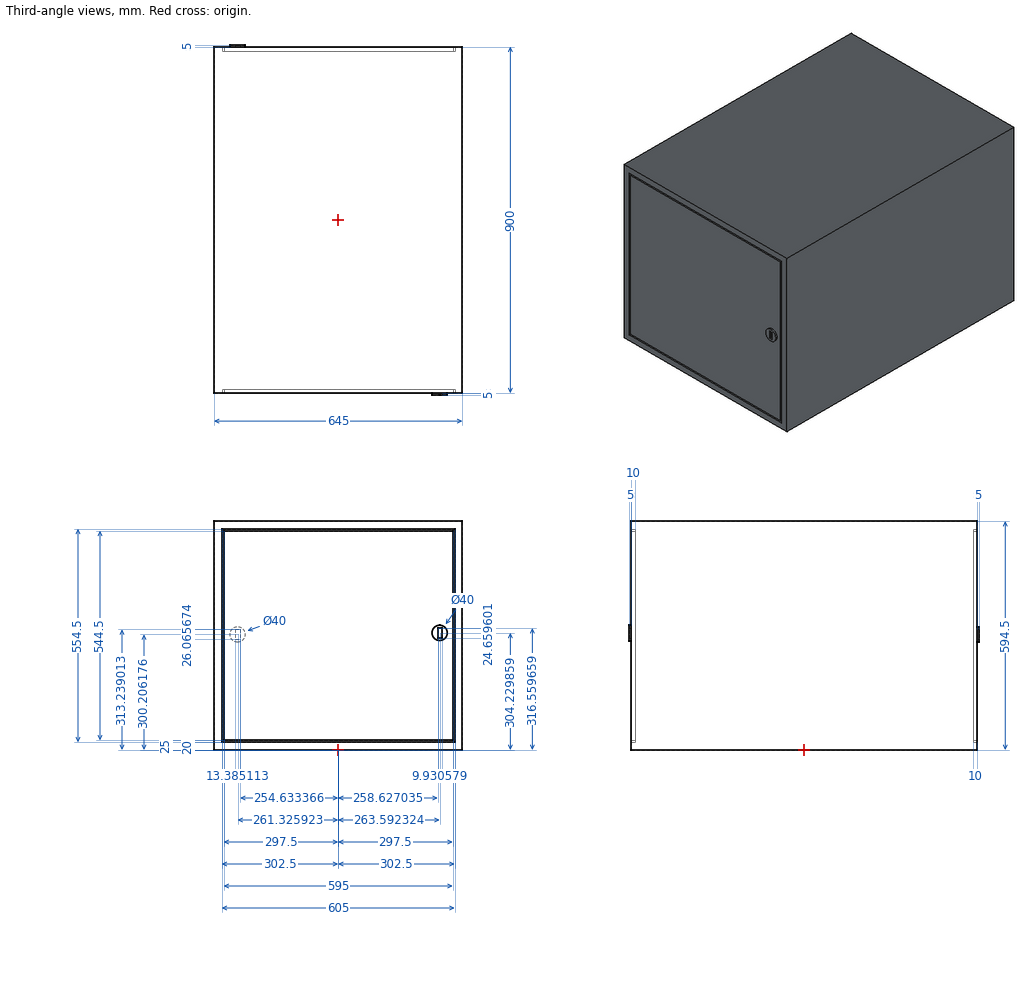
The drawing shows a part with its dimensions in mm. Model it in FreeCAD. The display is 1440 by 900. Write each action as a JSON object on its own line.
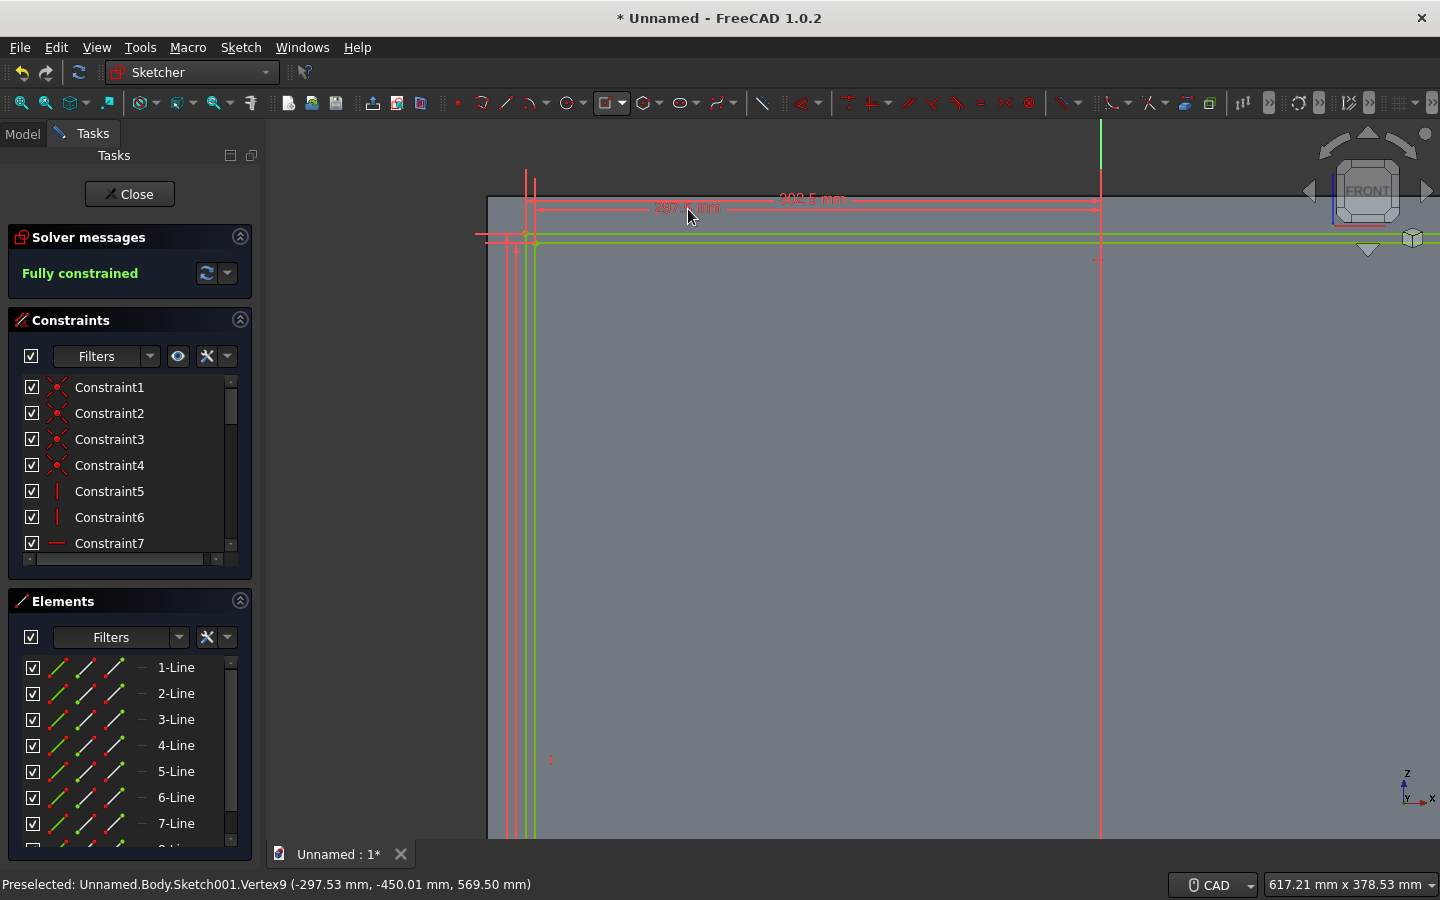
{"action": "left_click", "coordinate": [130, 194]}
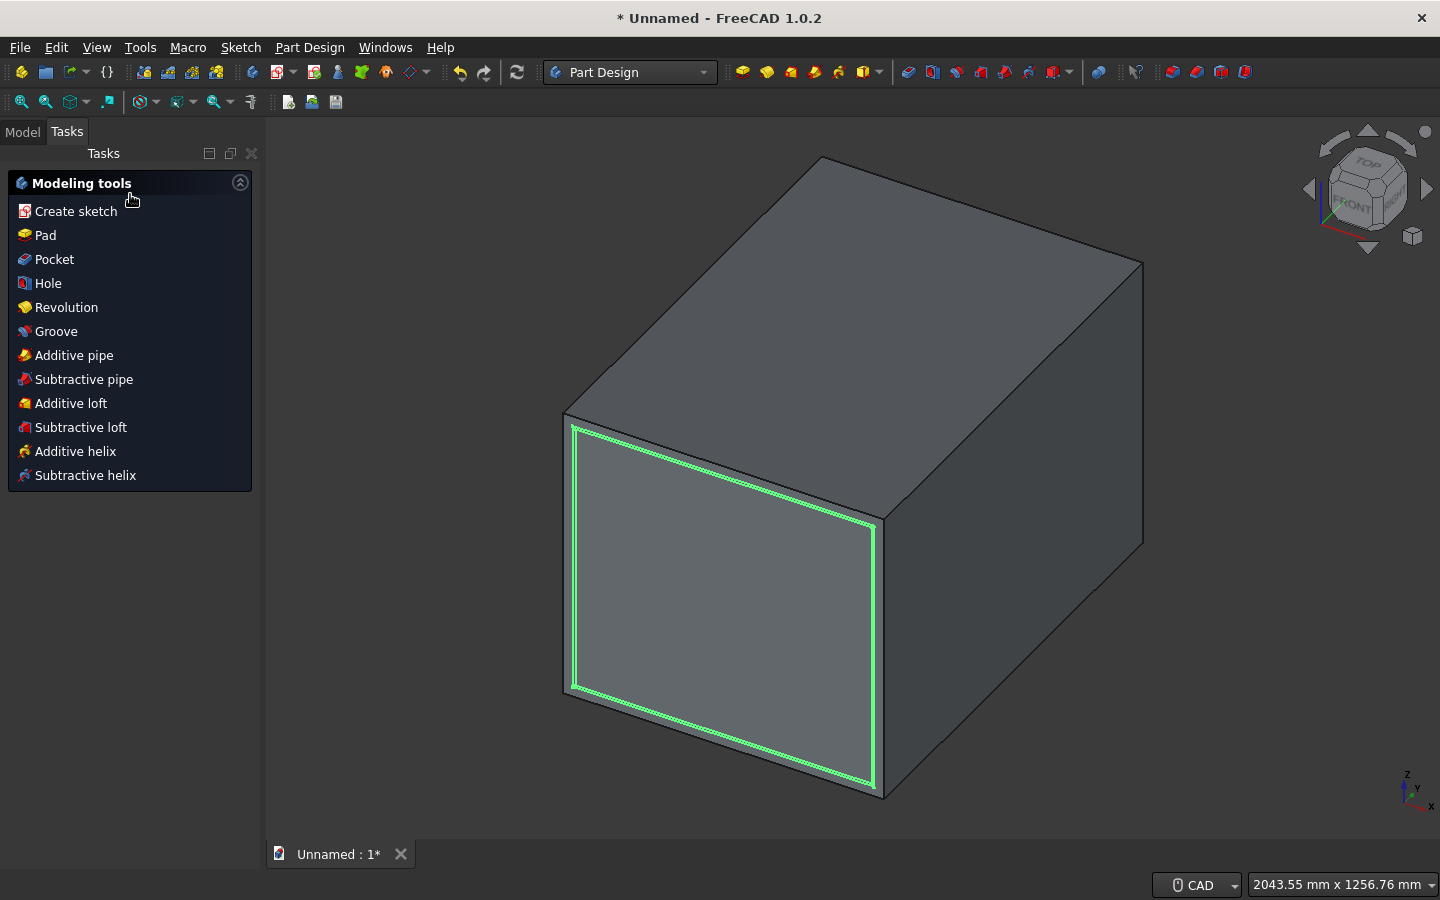
{"action": "left_click", "coordinate": [910, 72]}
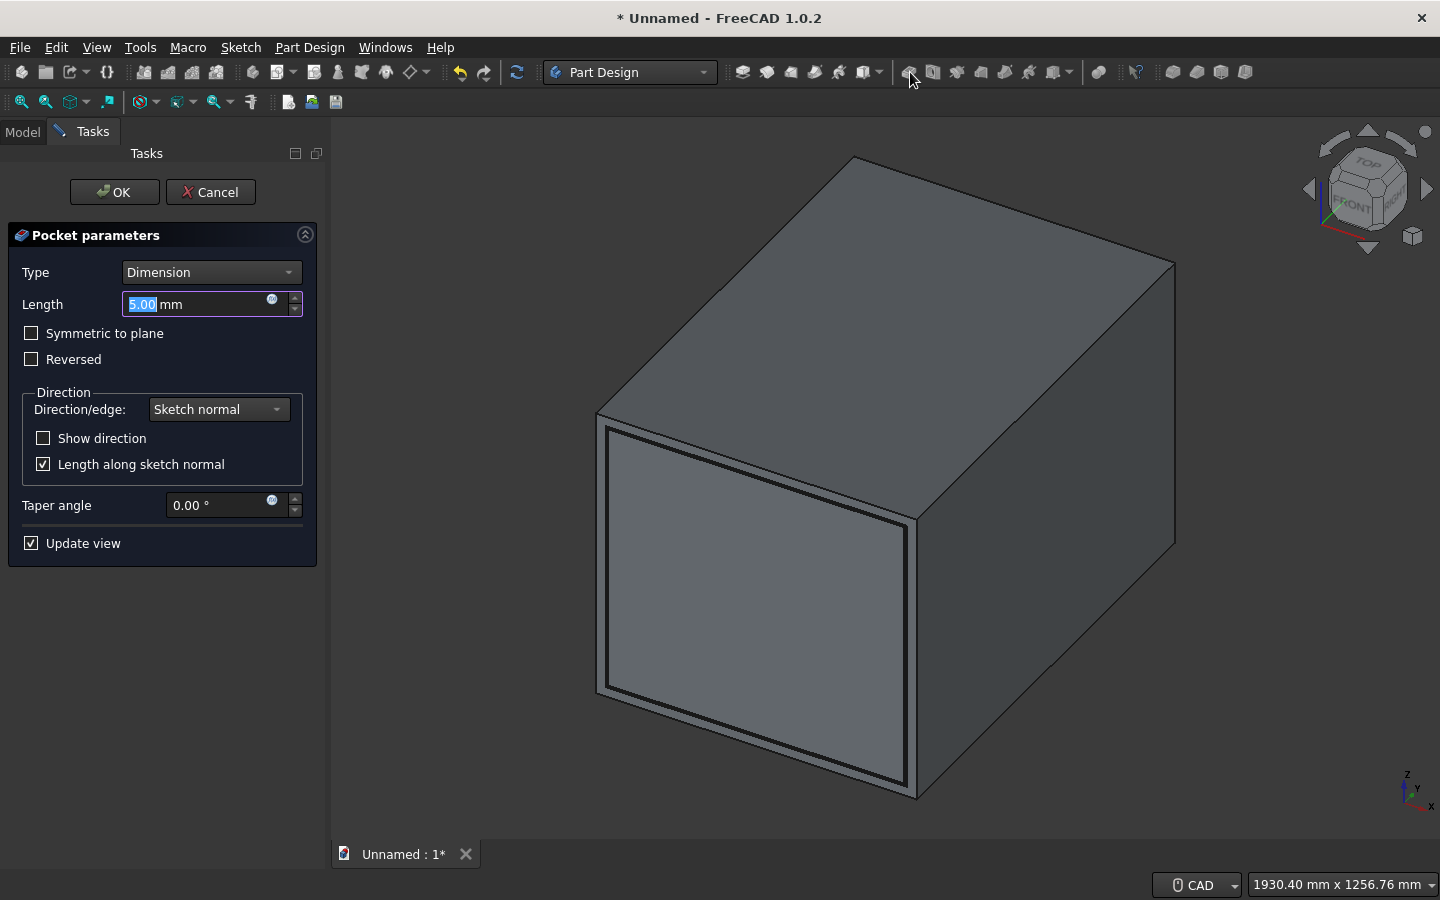
{"action": "type", "text": "10"}
{"action": "key", "text": "Tab"}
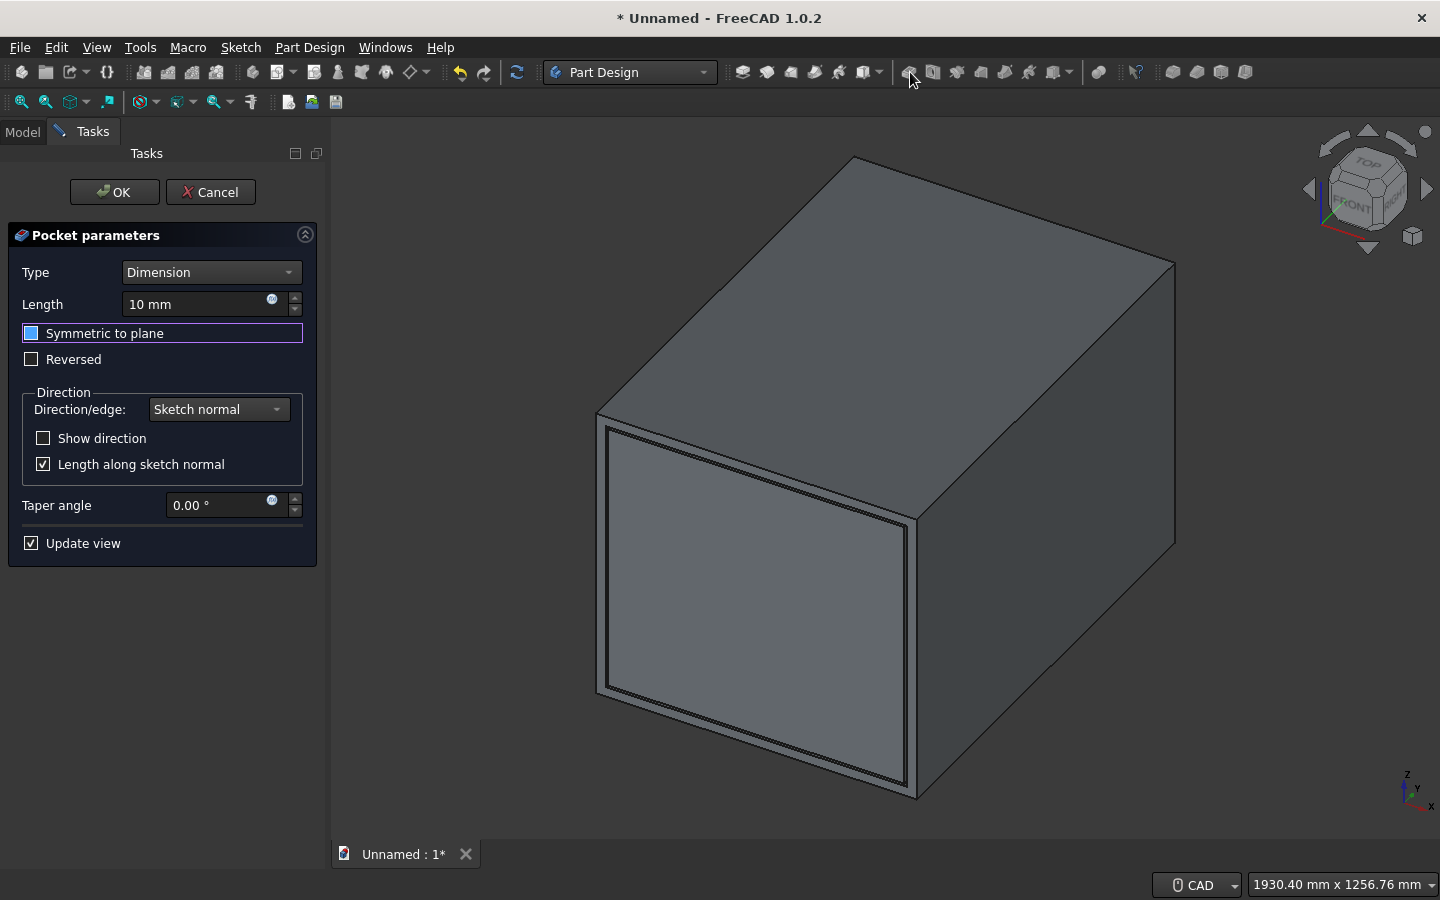
{"action": "left_click", "coordinate": [115, 192]}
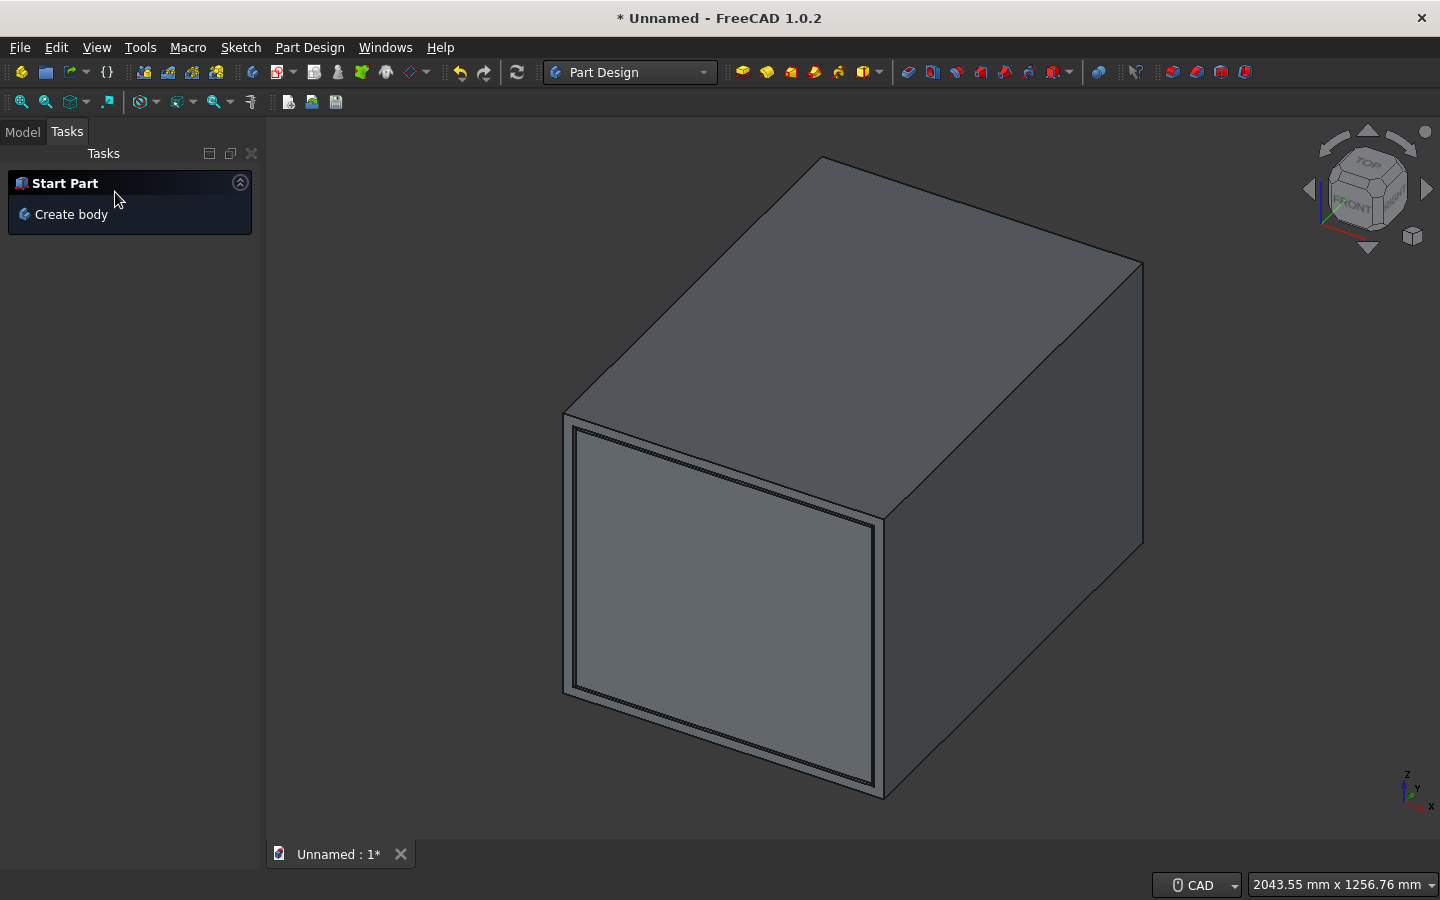
{"action": "left_click", "coordinate": [724, 605]}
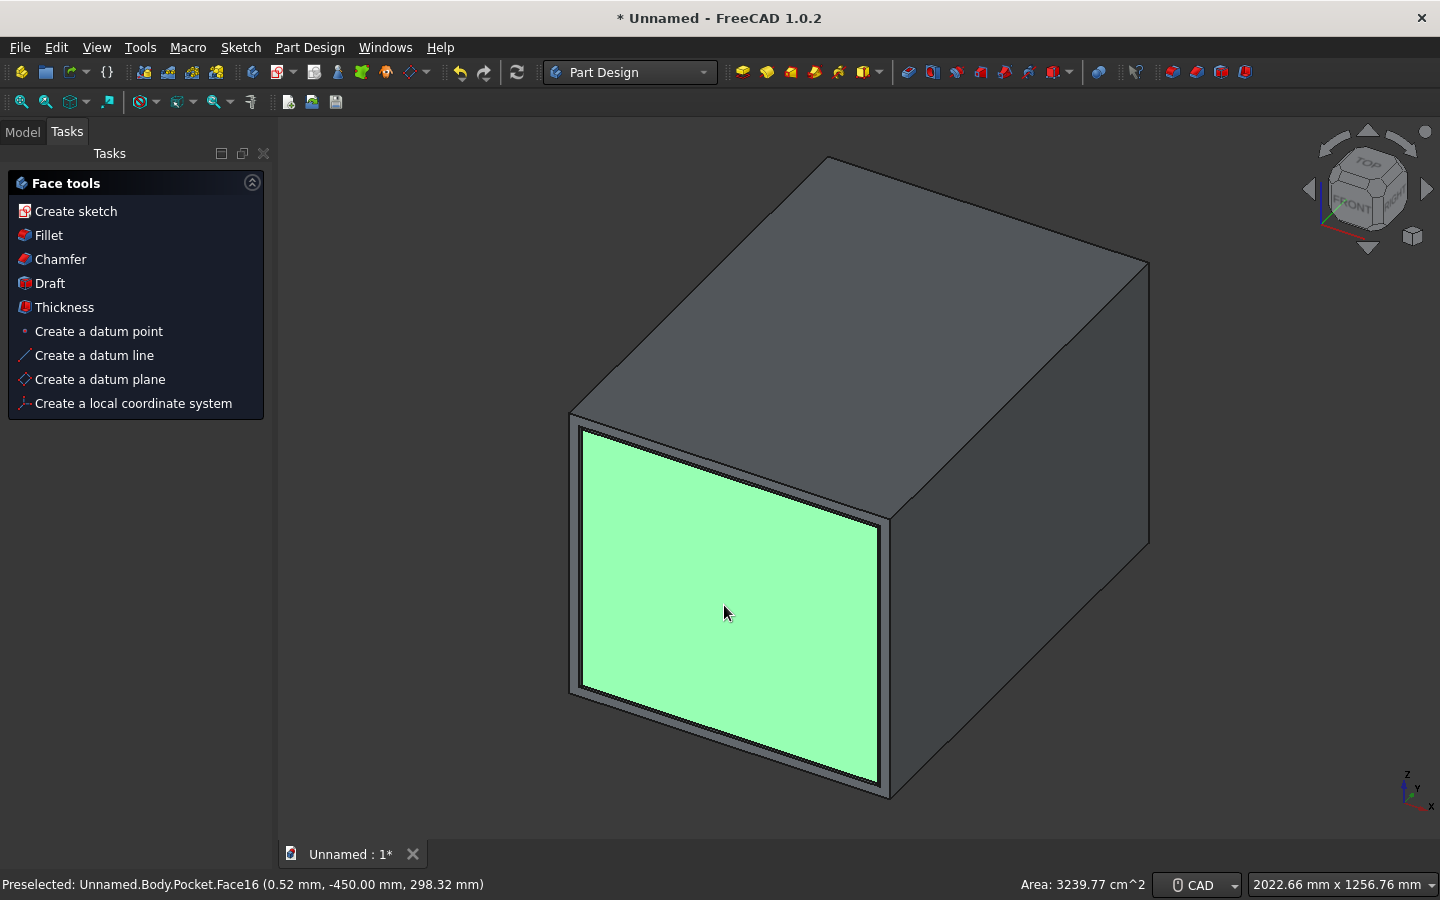
{"action": "left_click", "coordinate": [278, 72]}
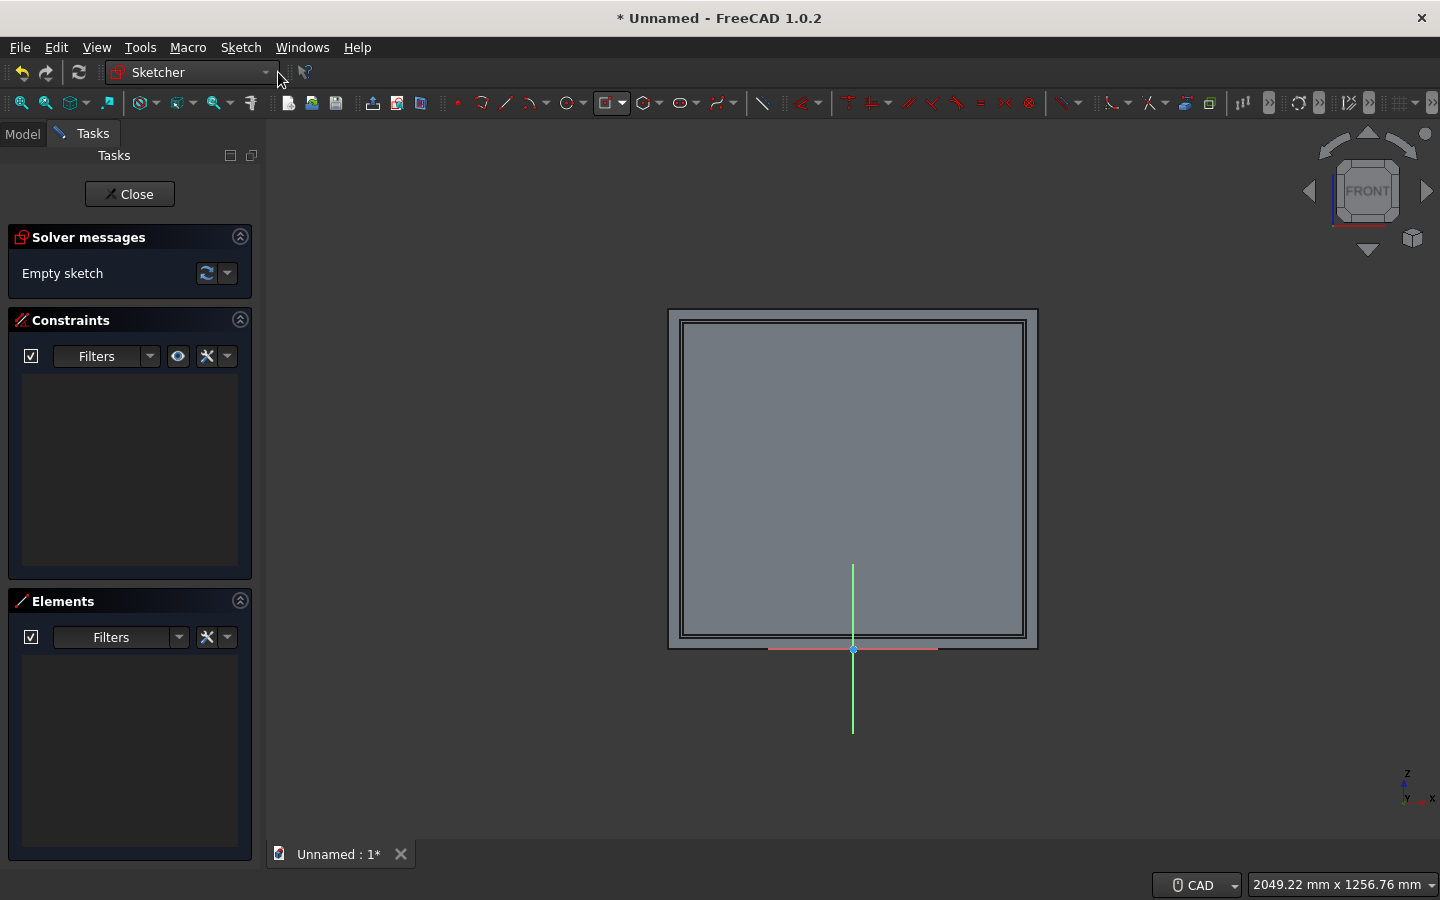
{"action": "scroll", "coordinate": [1016, 475], "scroll_direction": "up", "scroll_amount": 15}